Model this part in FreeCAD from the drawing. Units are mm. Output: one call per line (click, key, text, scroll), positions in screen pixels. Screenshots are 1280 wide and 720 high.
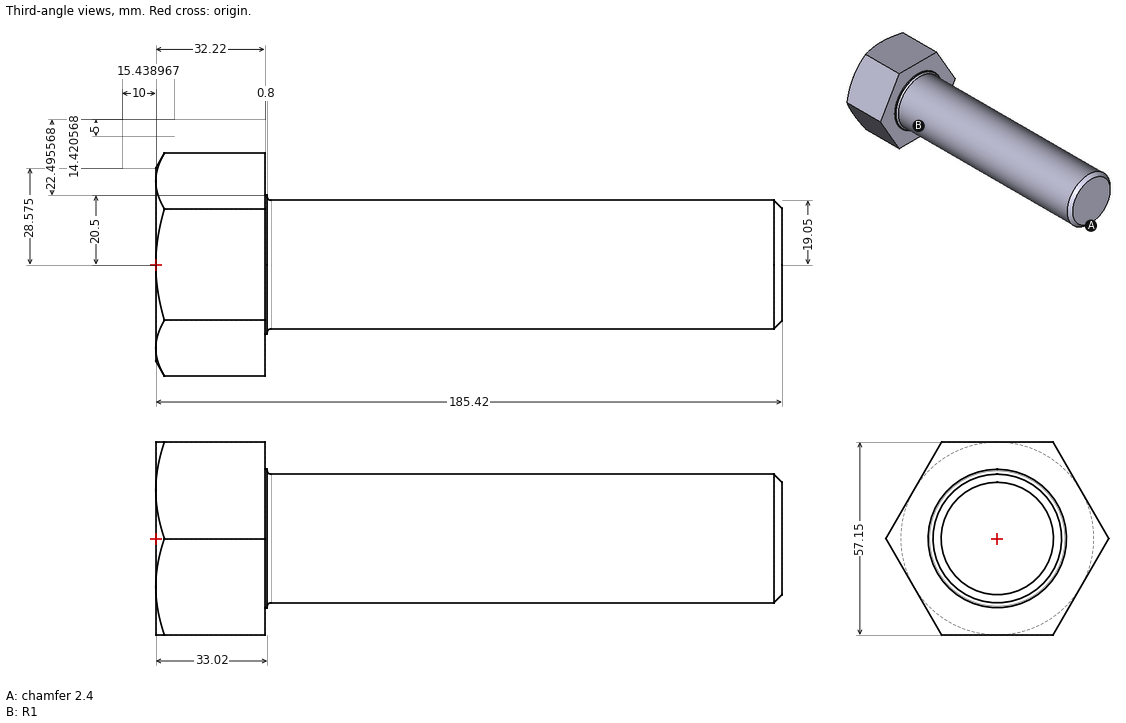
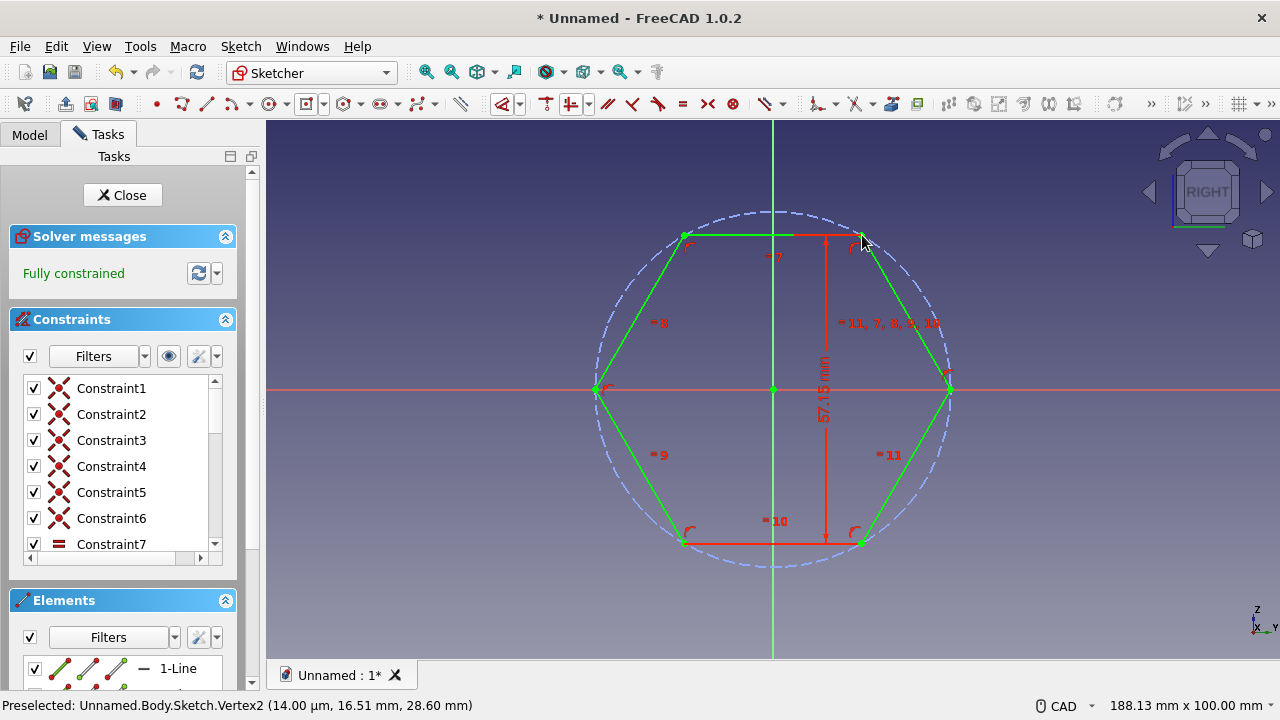
click(123, 195)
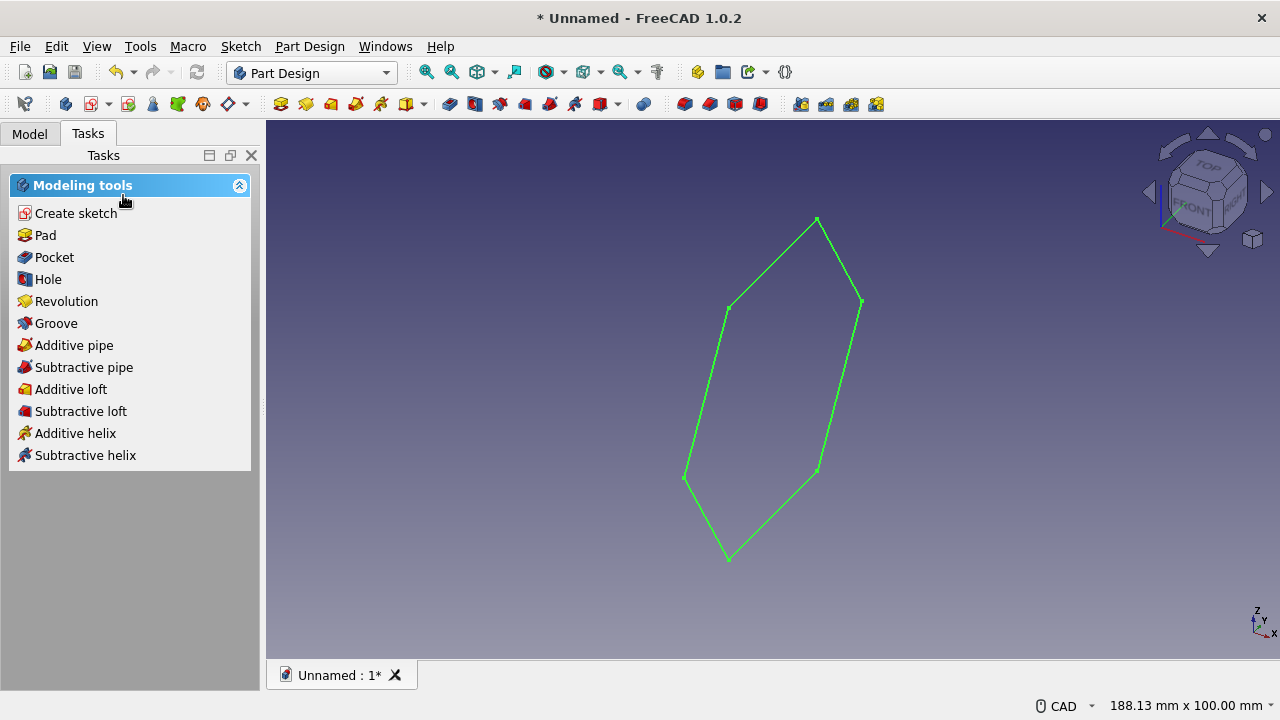
click(281, 104)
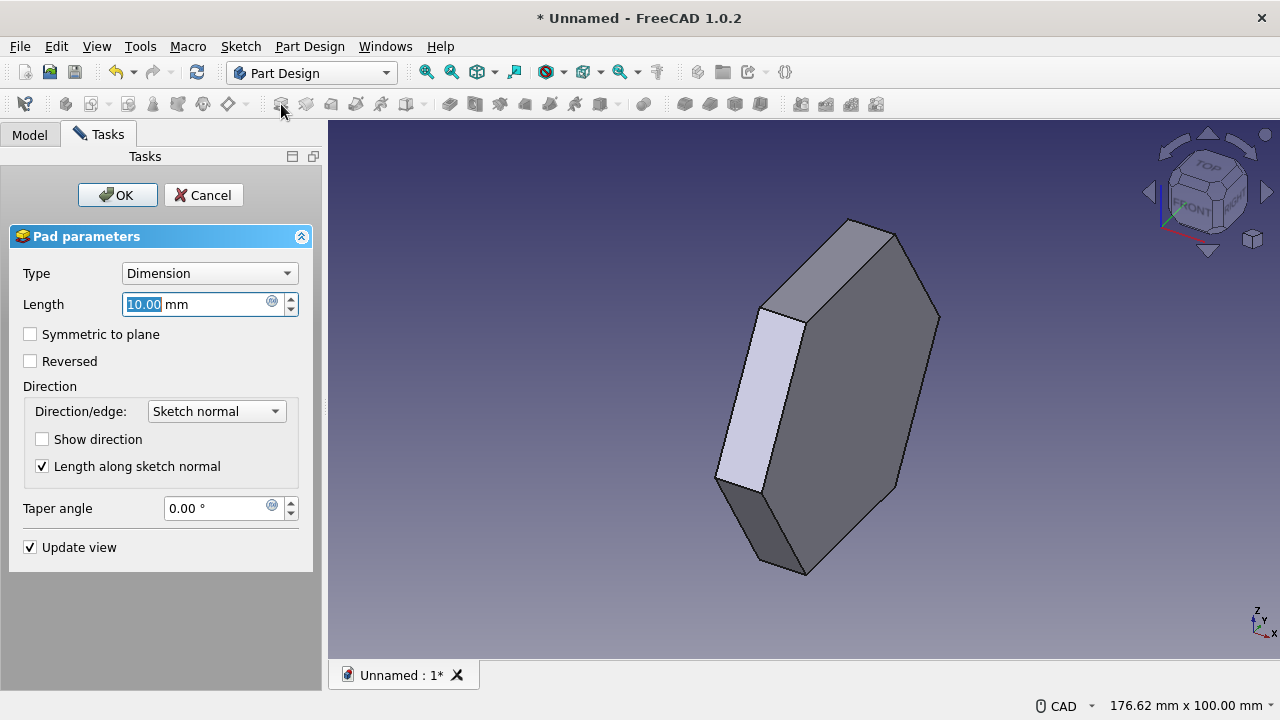
text(33.02)
key(Tab)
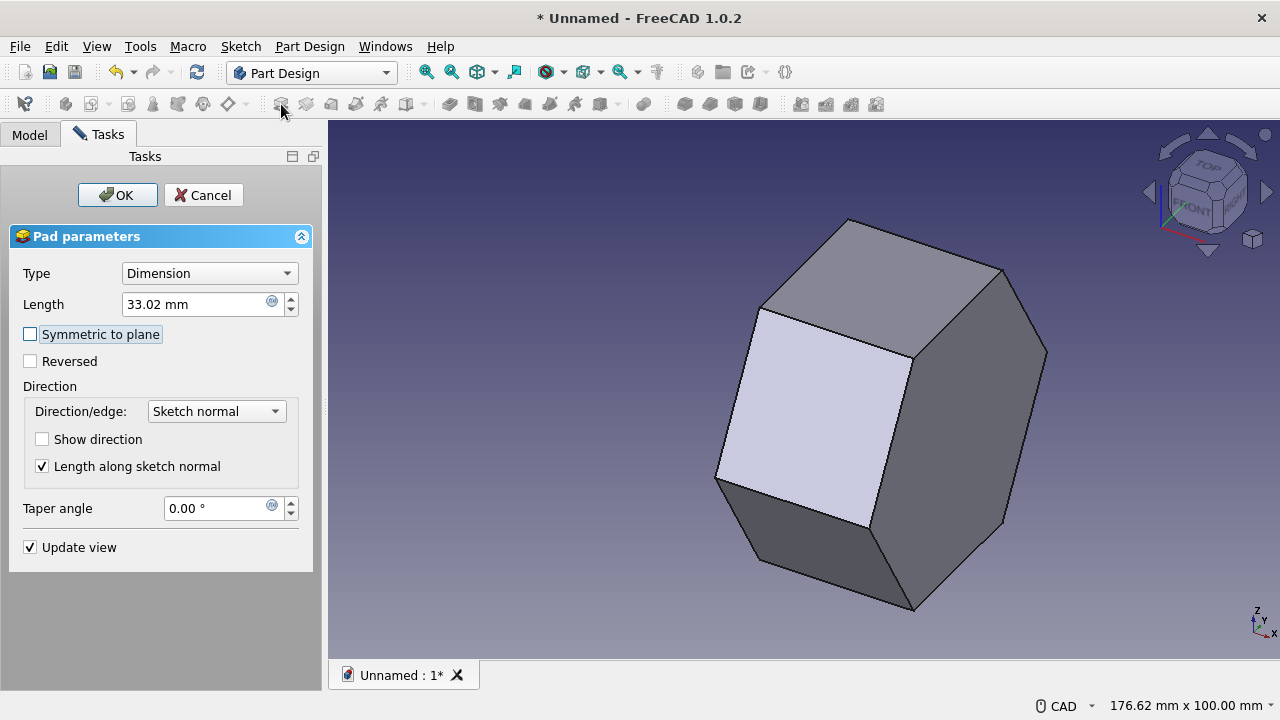
click(118, 195)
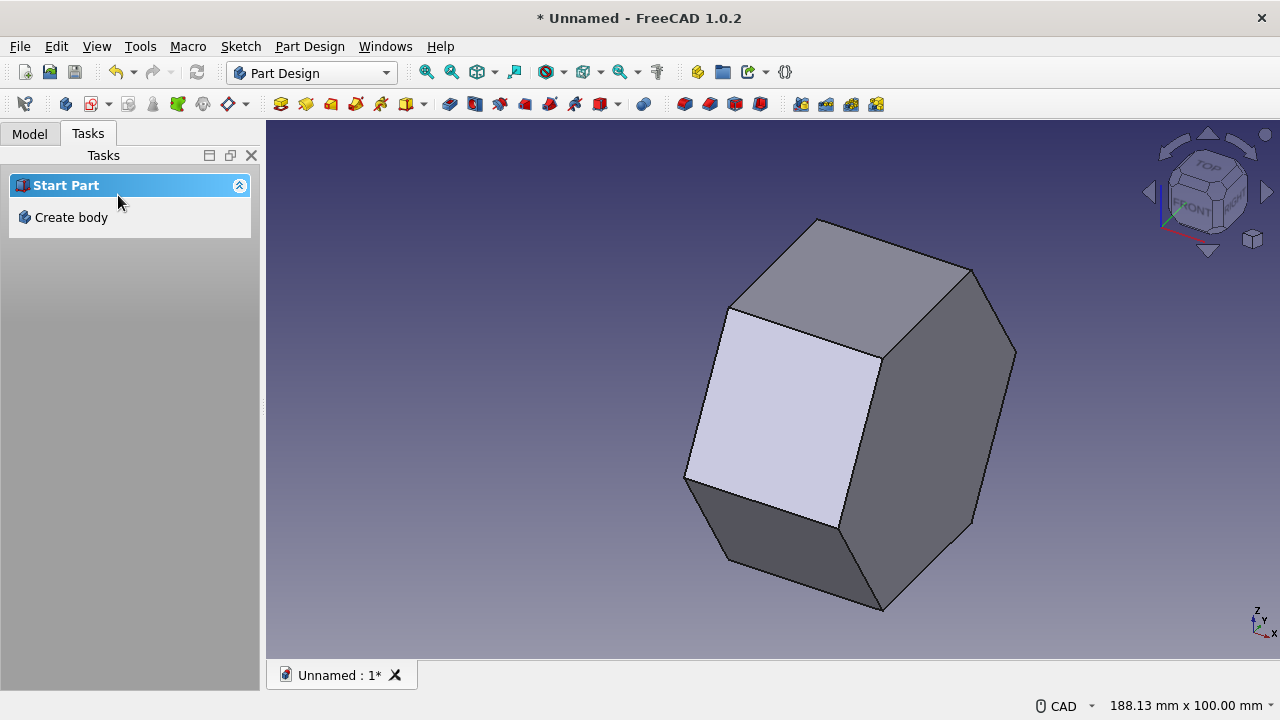
click(90, 104)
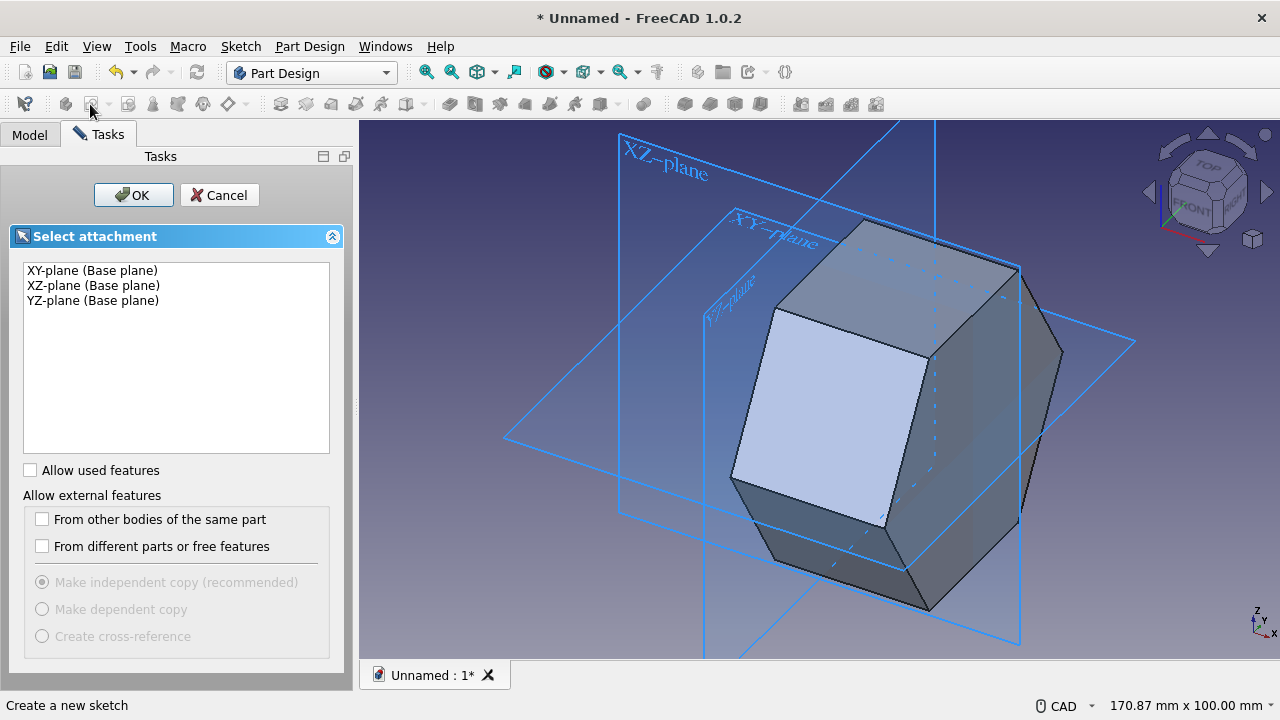
click(84, 270)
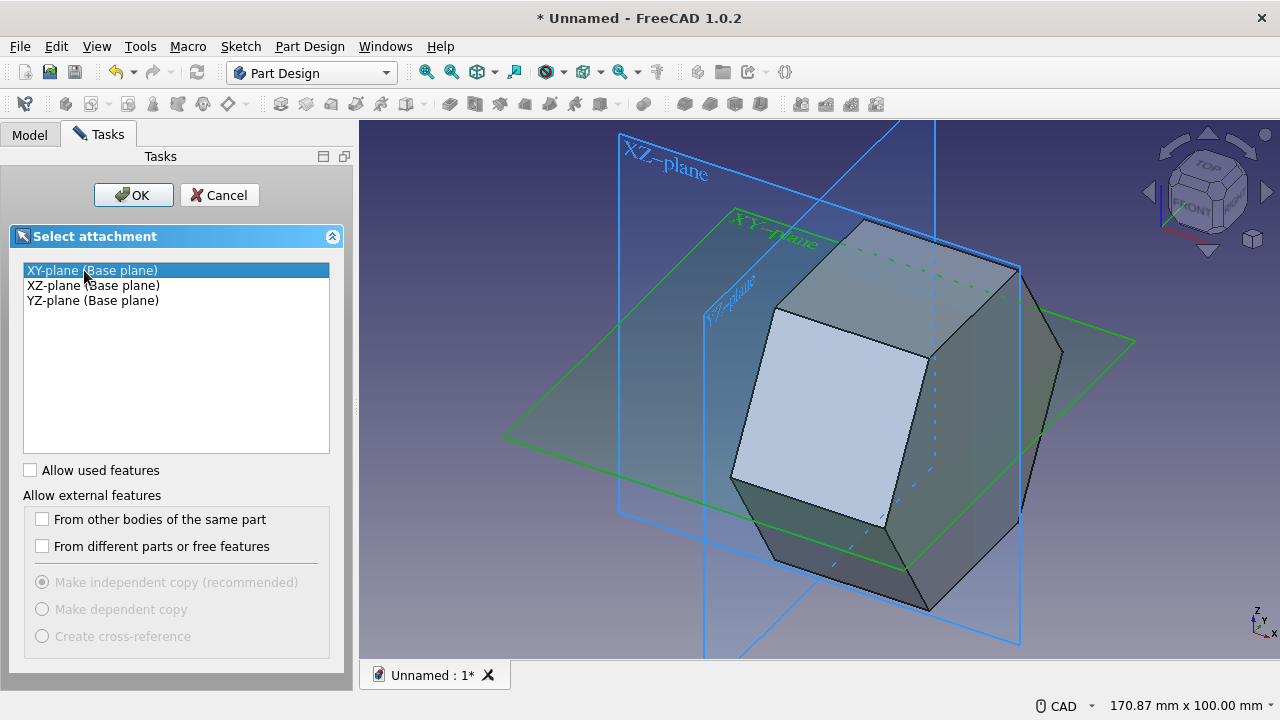
click(134, 195)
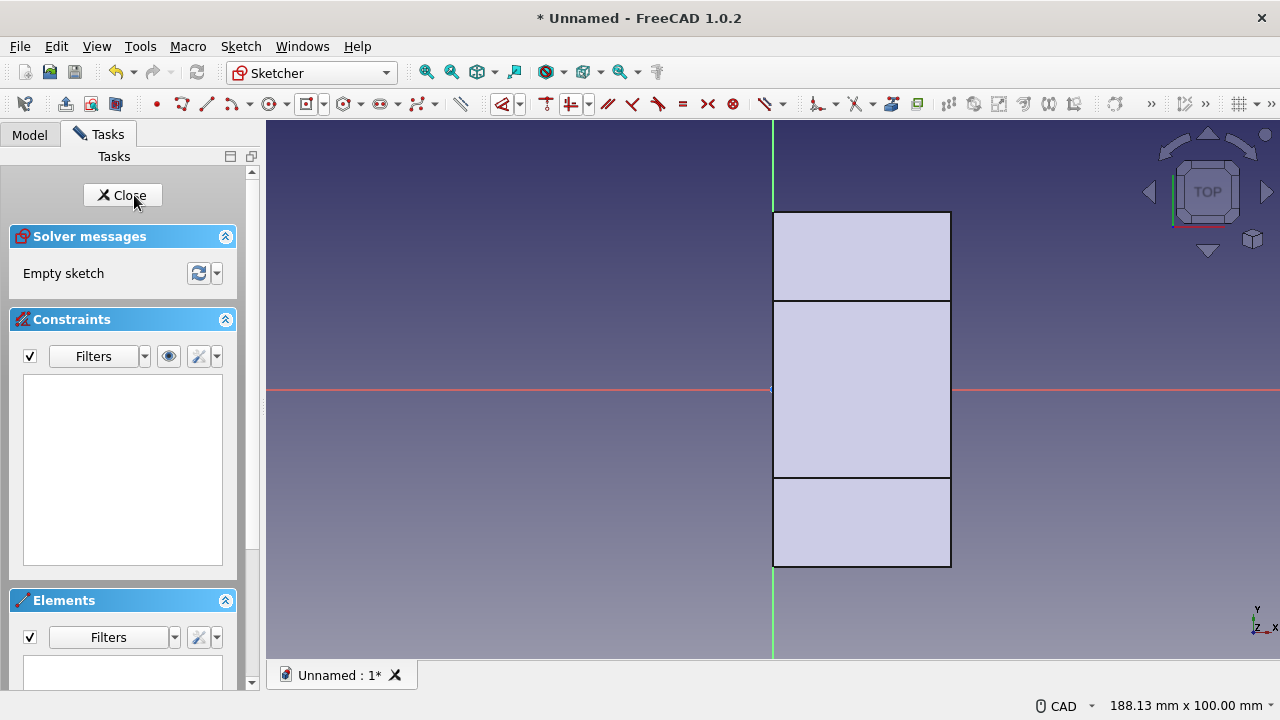
click(116, 104)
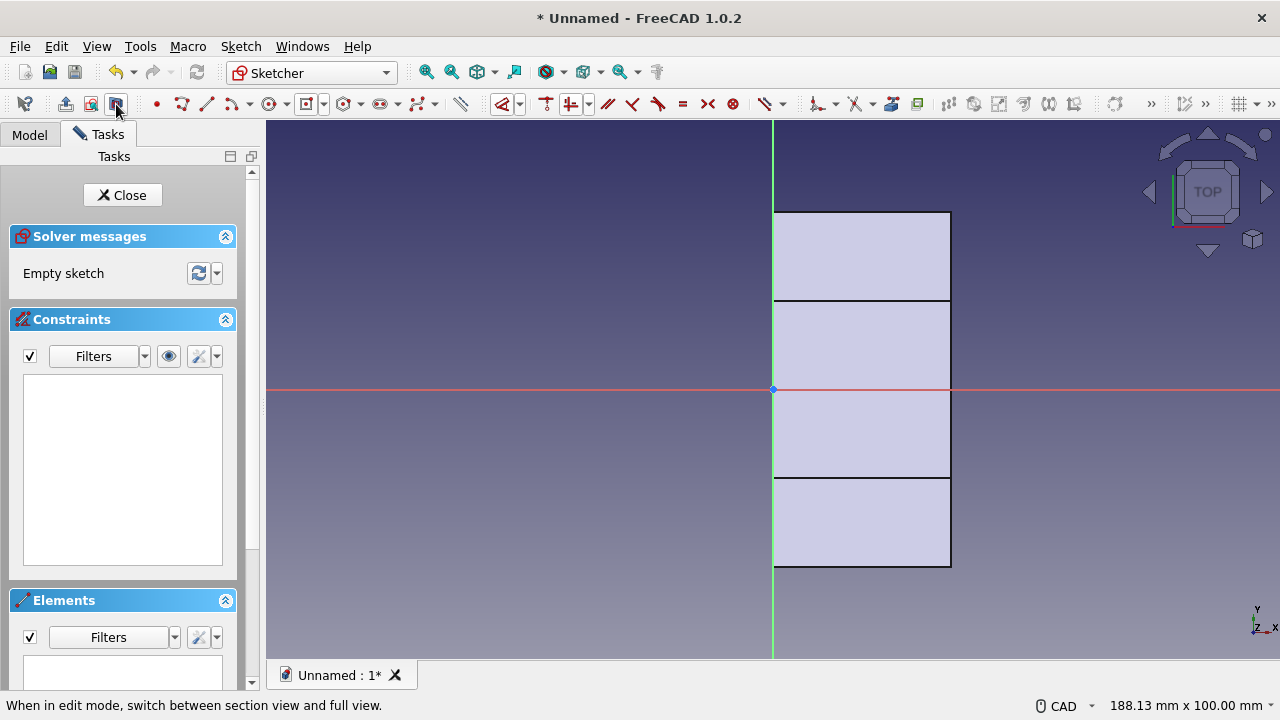
scroll(294, 431, down, 4)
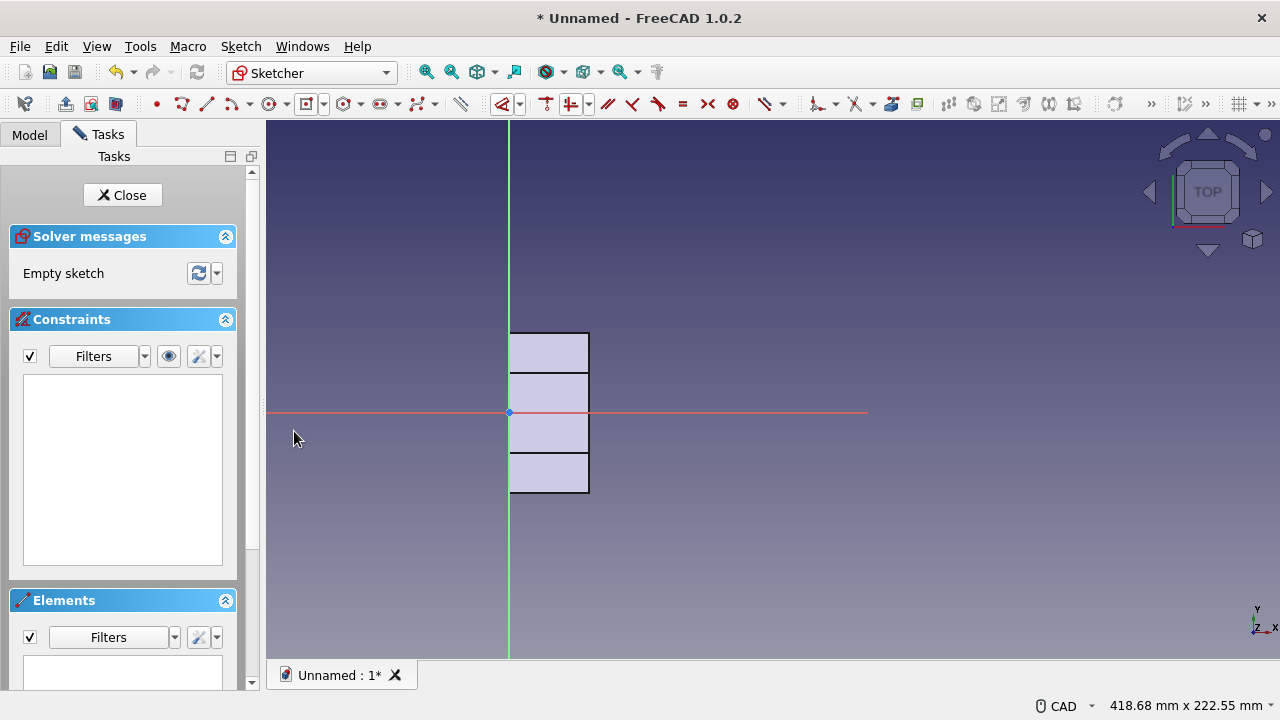
key(g)
key(r)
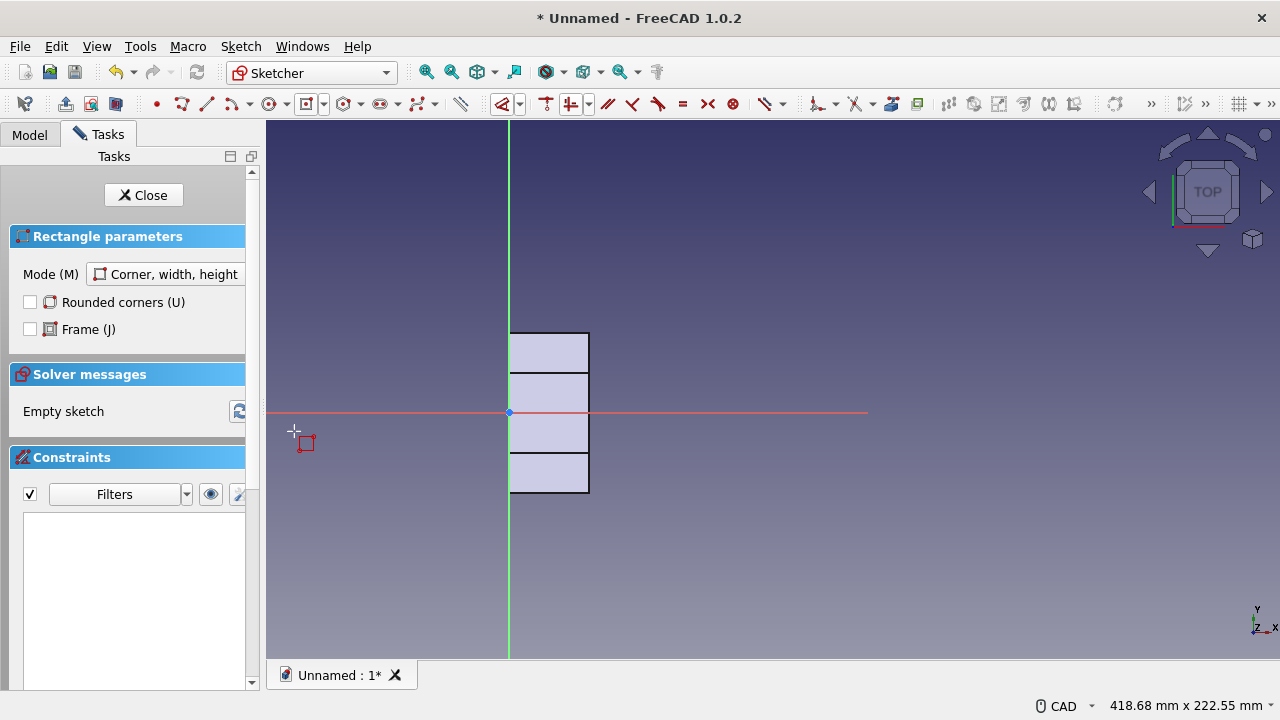
click(509, 413)
move(958, 367)